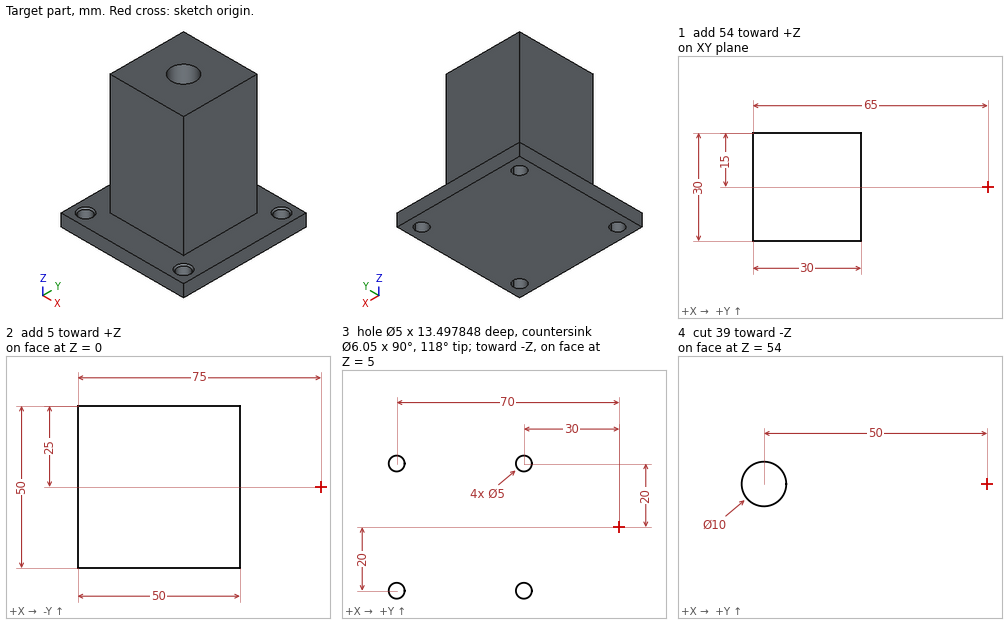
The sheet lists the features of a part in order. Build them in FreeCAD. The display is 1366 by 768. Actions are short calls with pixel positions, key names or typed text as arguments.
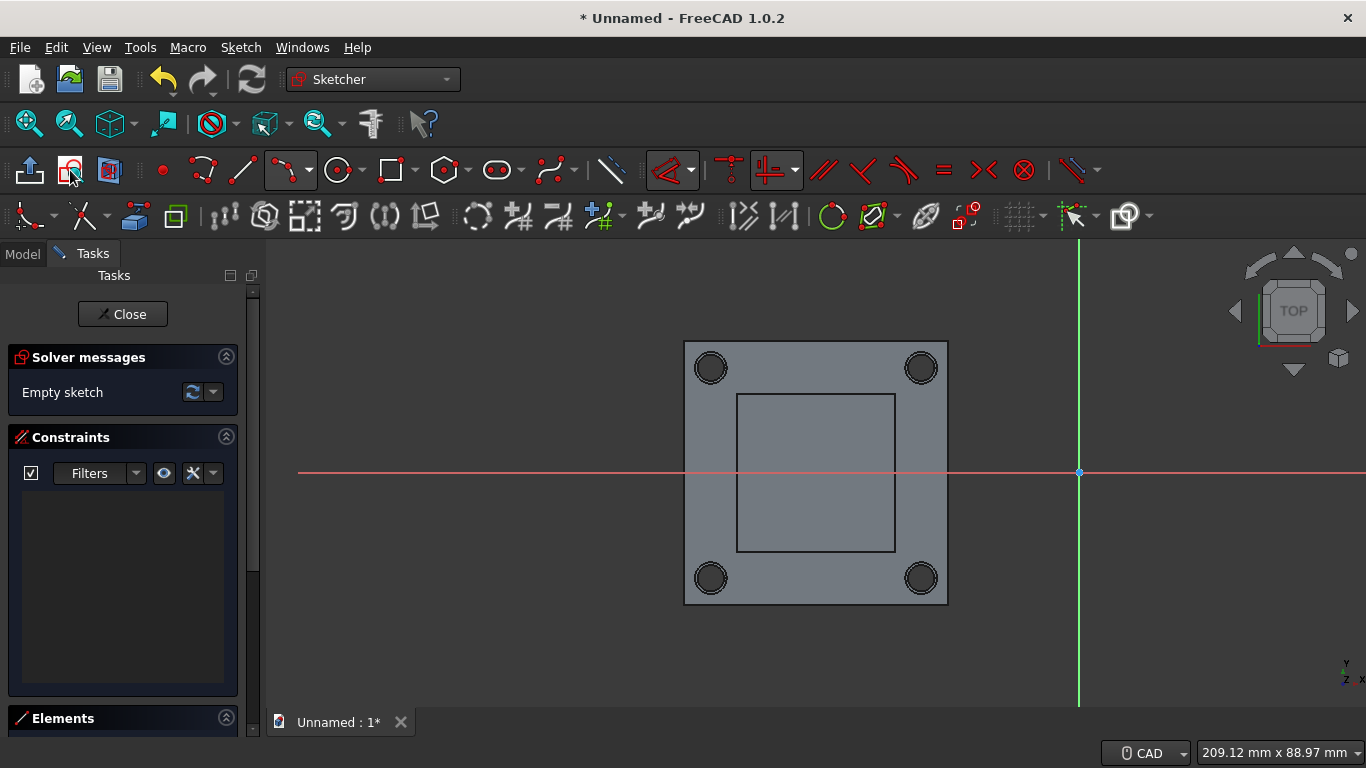
scroll(830, 473, up, 9)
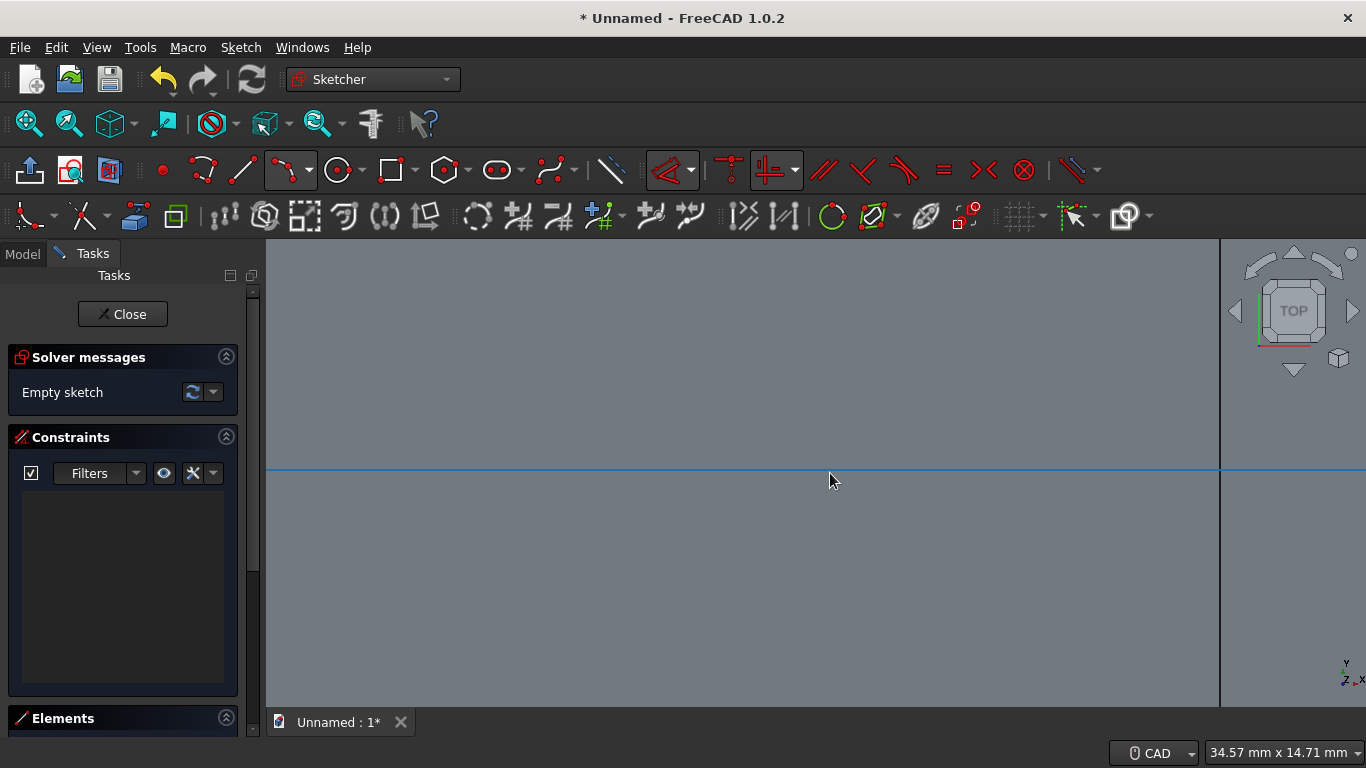
key(g)
key(c)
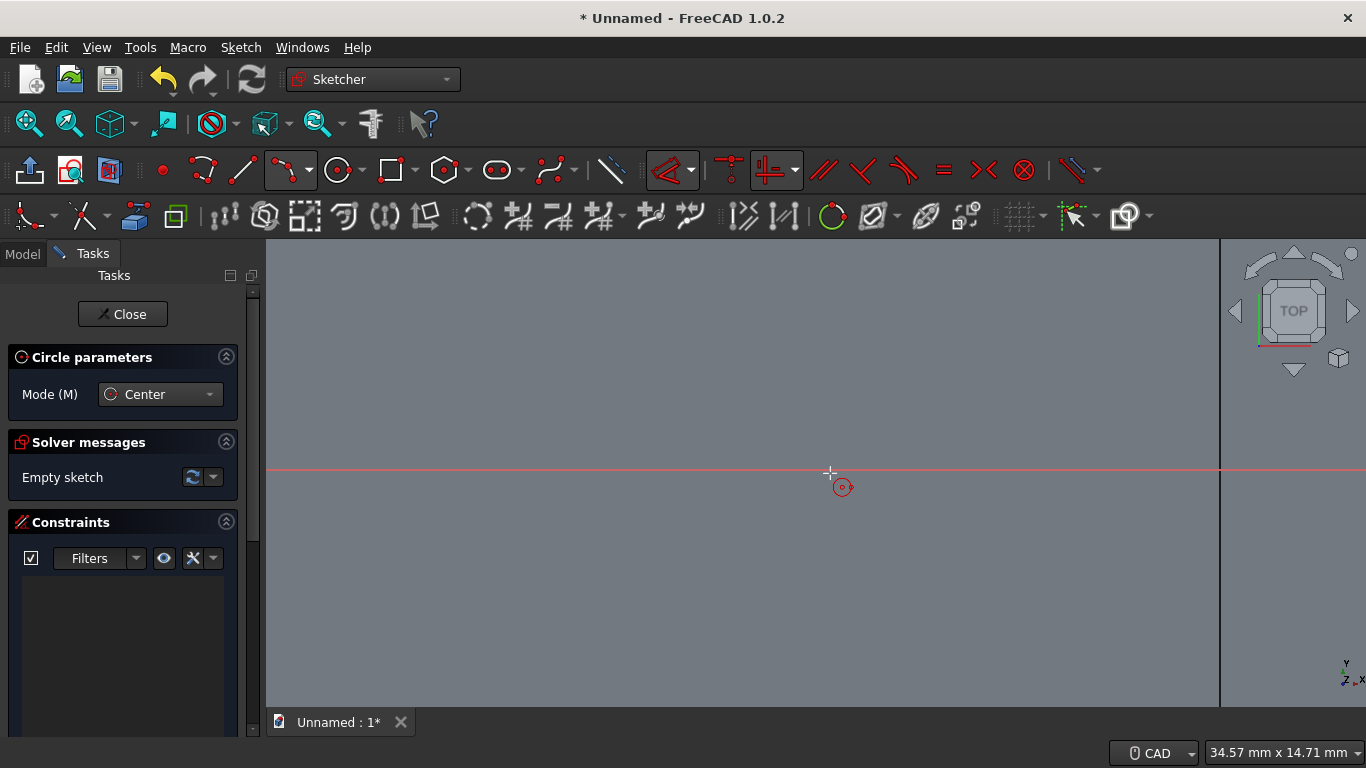
click(743, 470)
click(855, 358)
key(Escape)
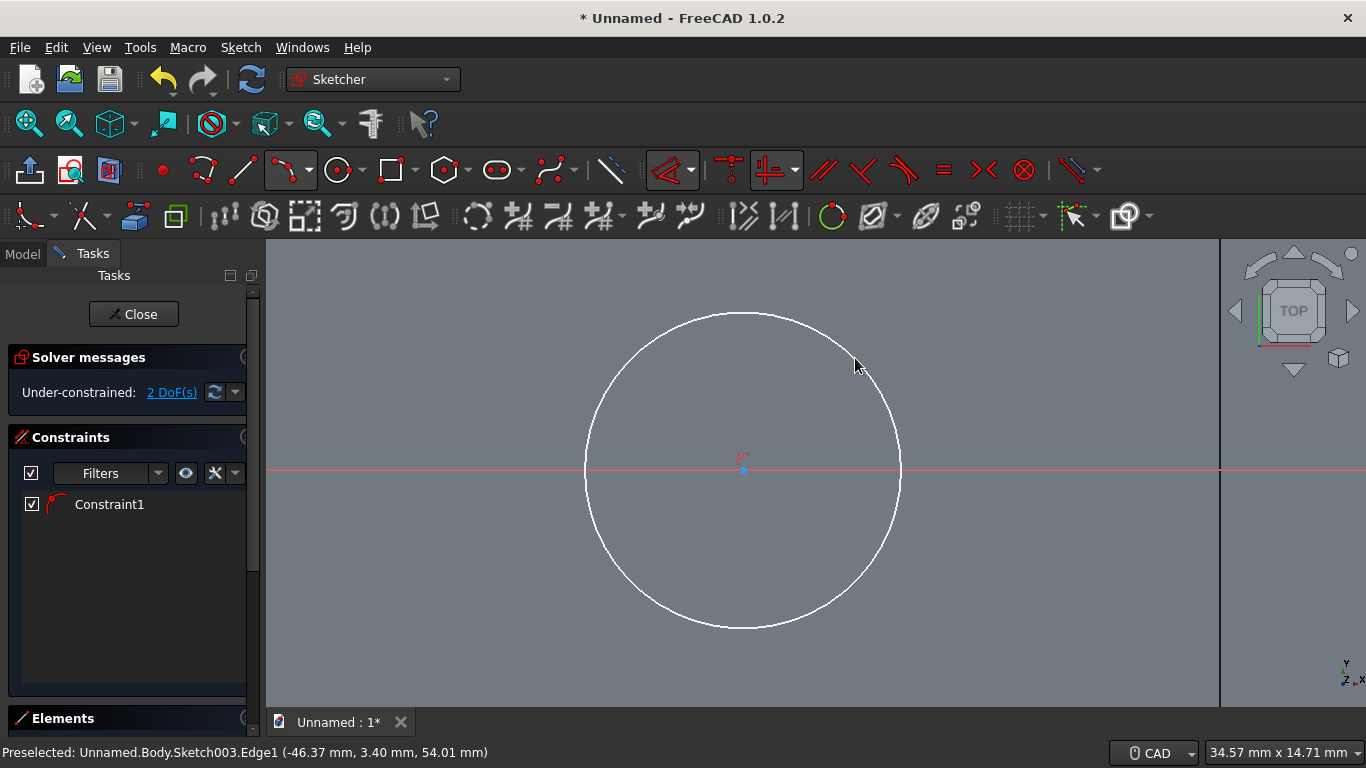
key(d)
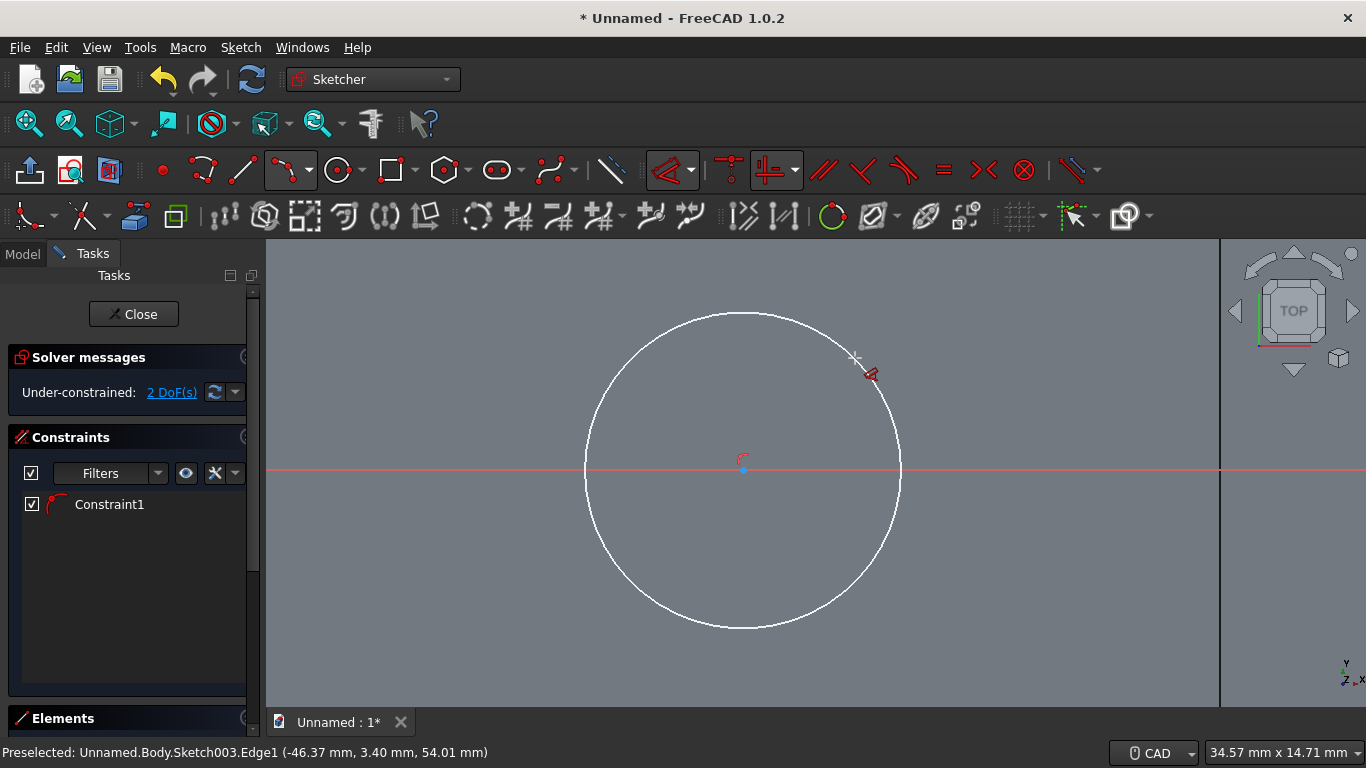
click(854, 358)
click(876, 335)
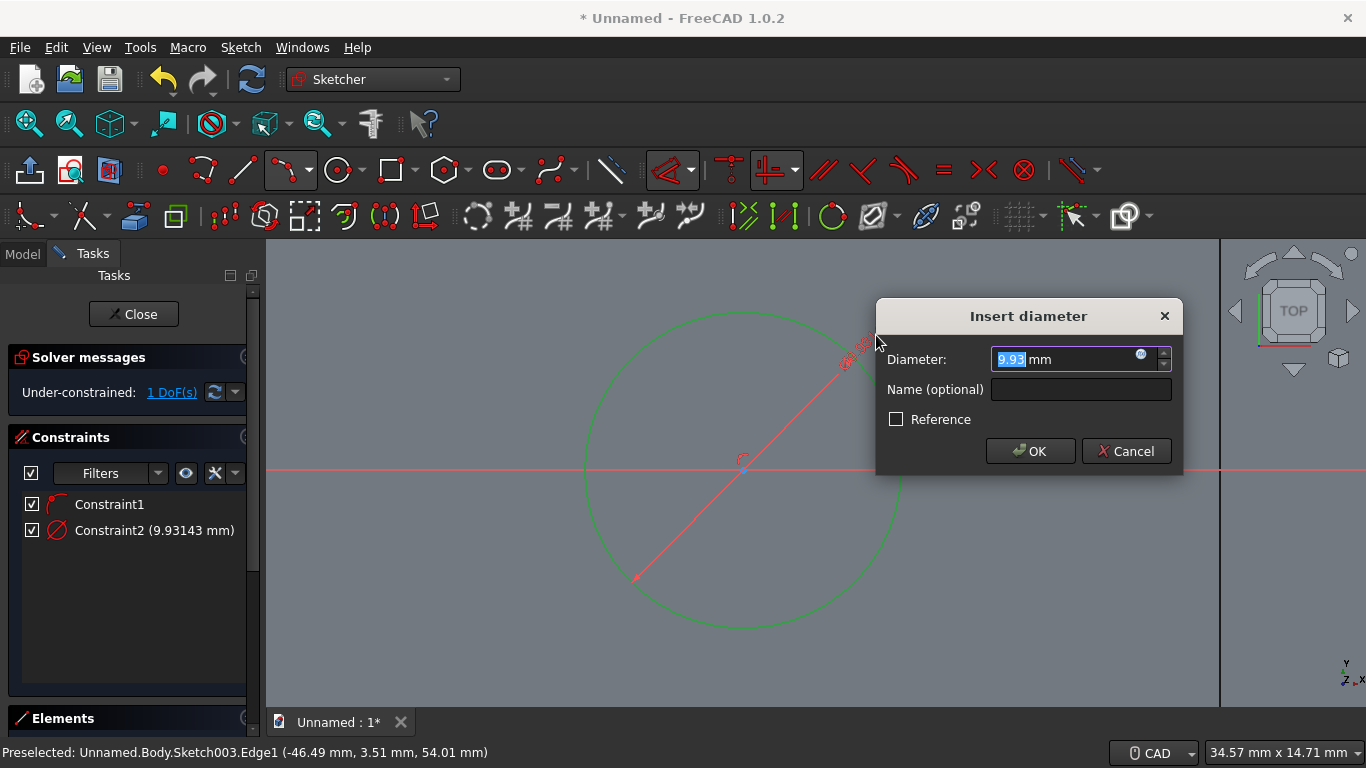
text(10)
key(Return)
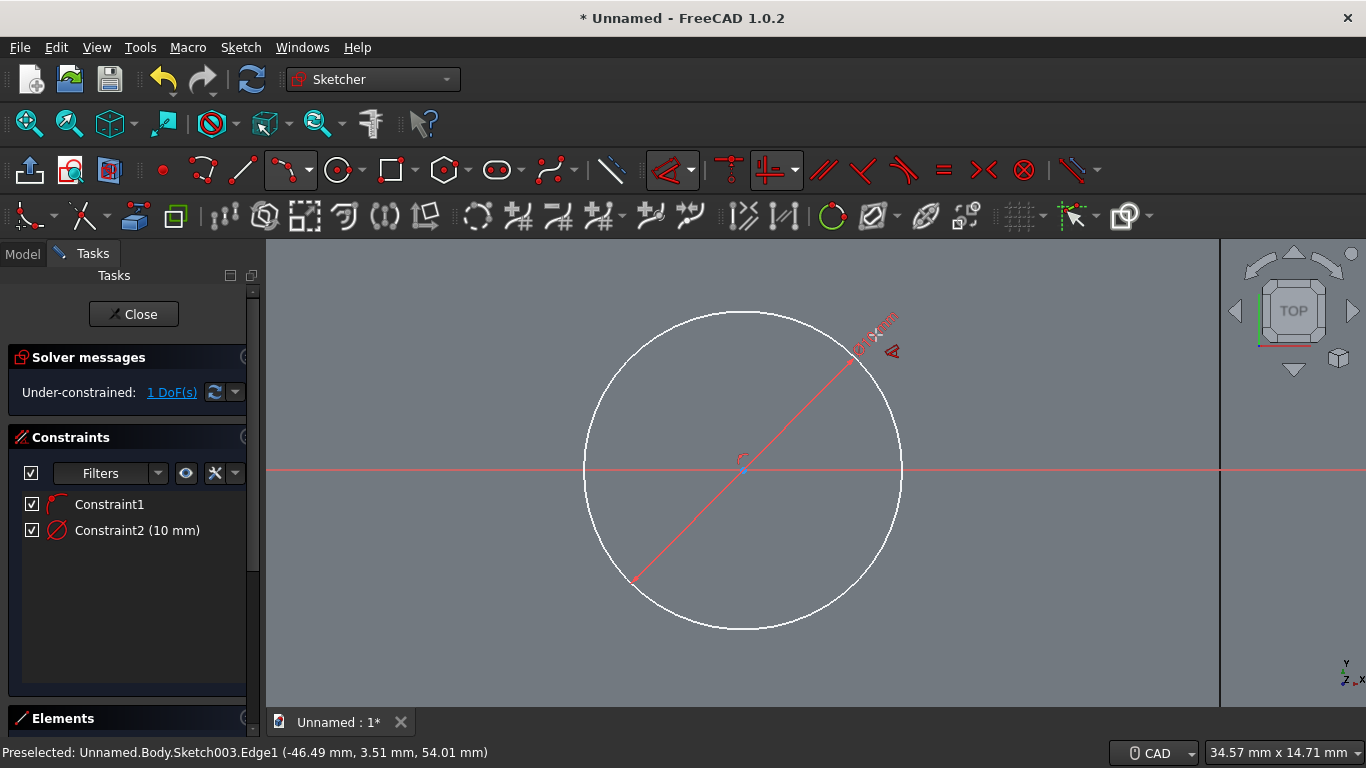
click(743, 470)
click(972, 504)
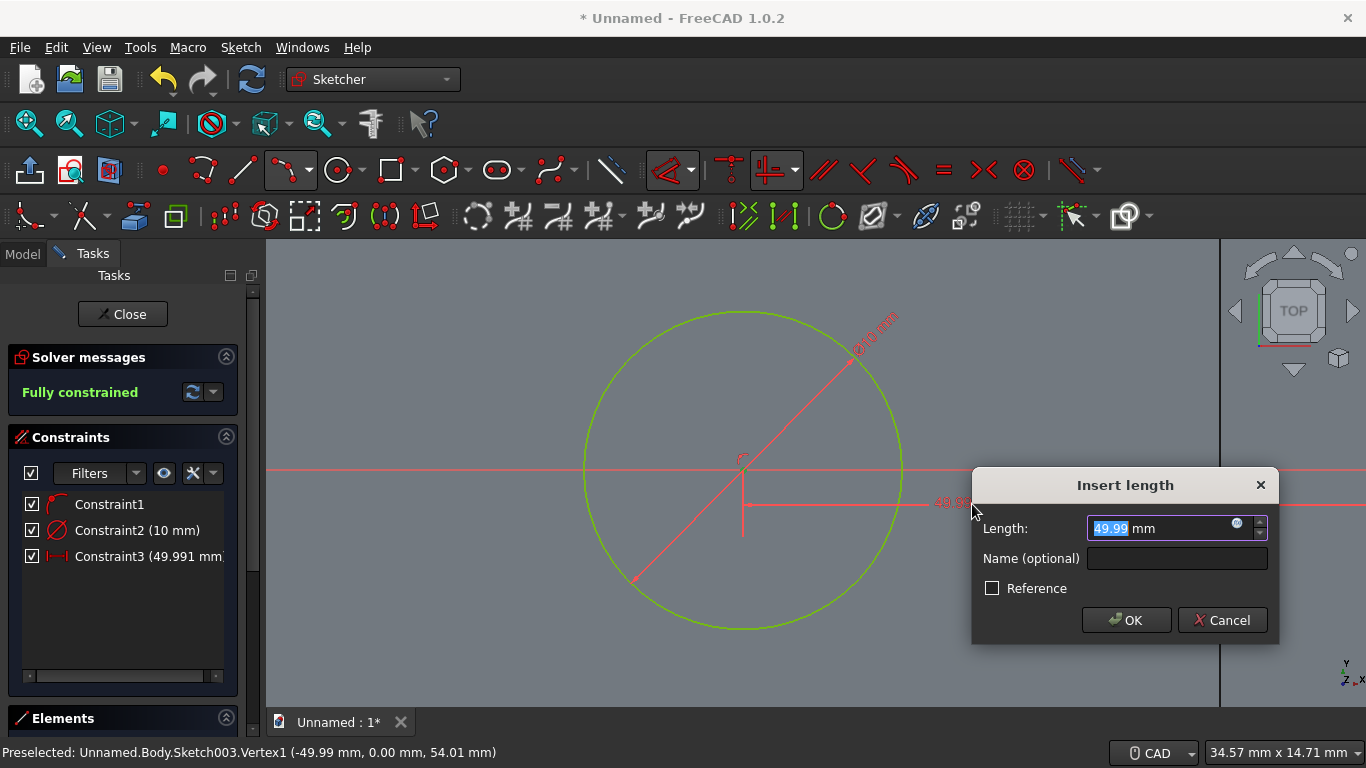
text(50)
key(Return)
key(Escape)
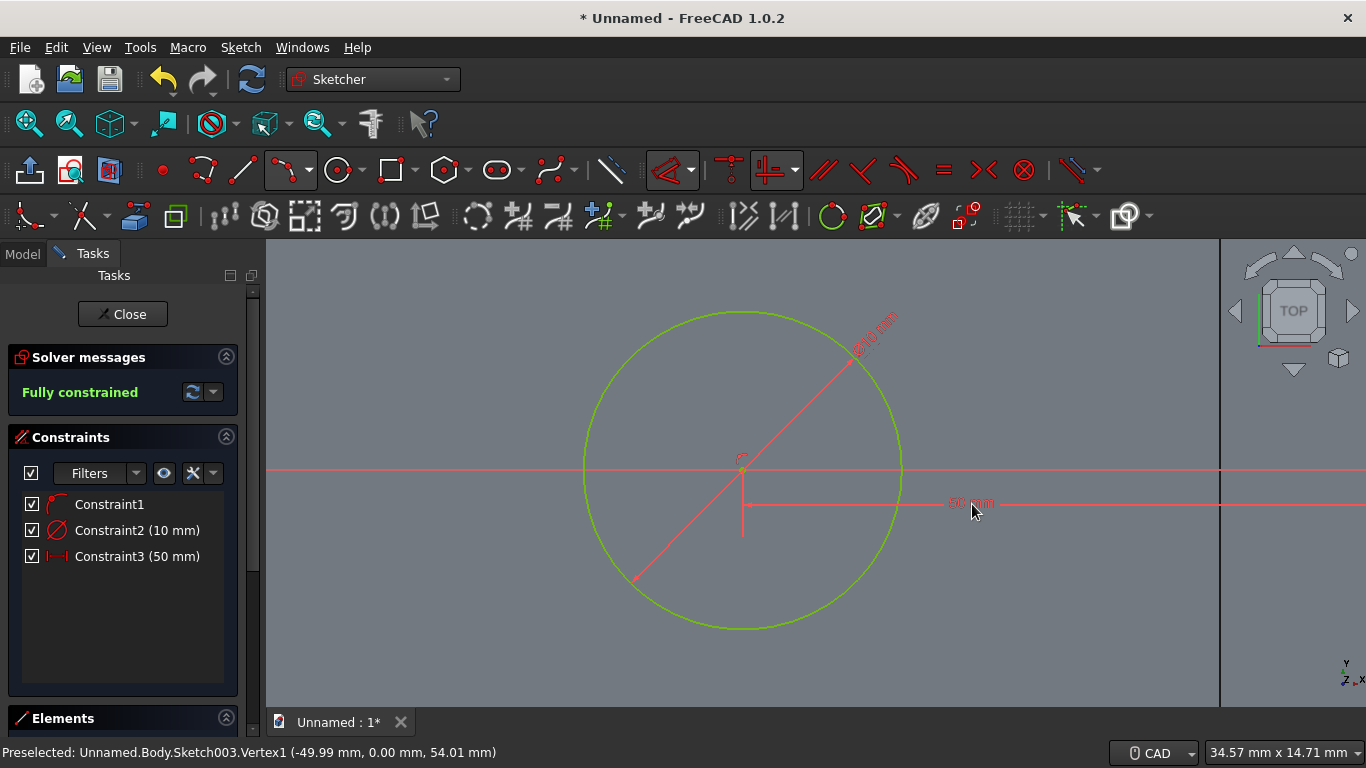
click(123, 314)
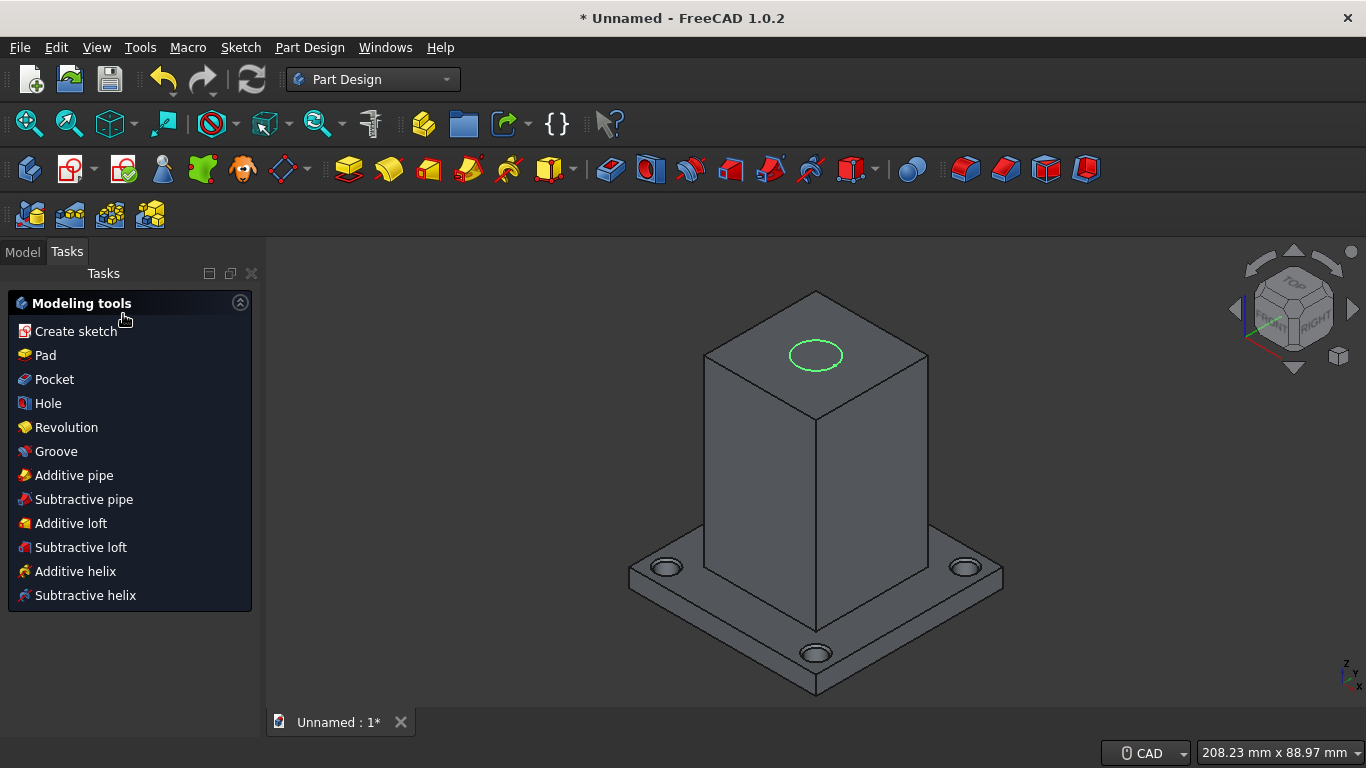
click(612, 170)